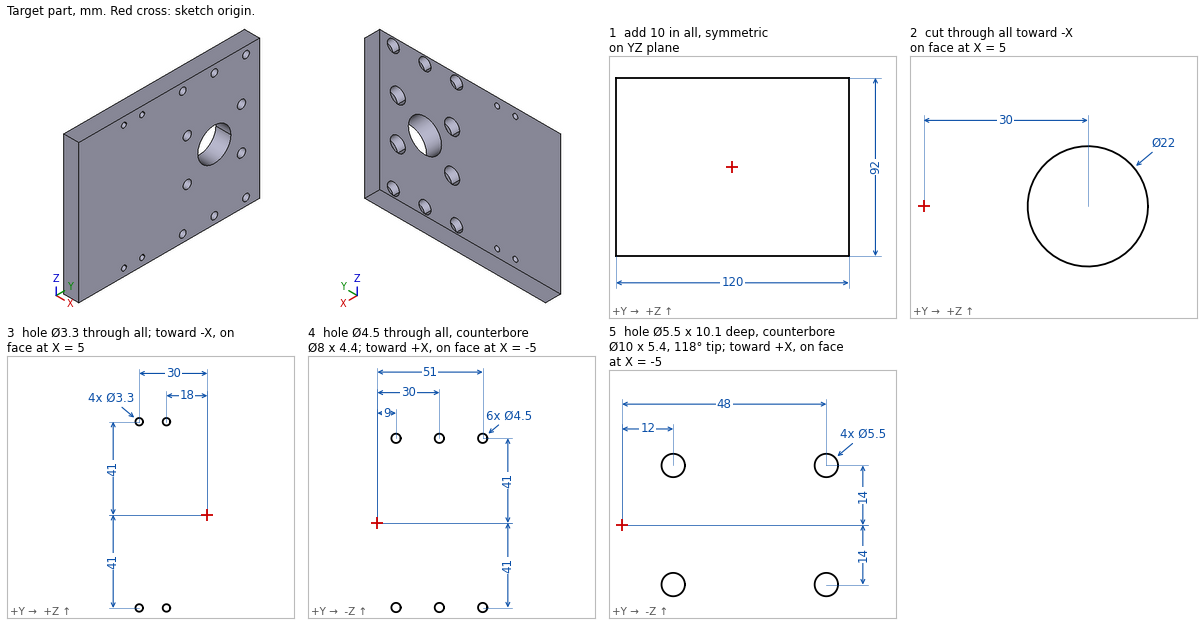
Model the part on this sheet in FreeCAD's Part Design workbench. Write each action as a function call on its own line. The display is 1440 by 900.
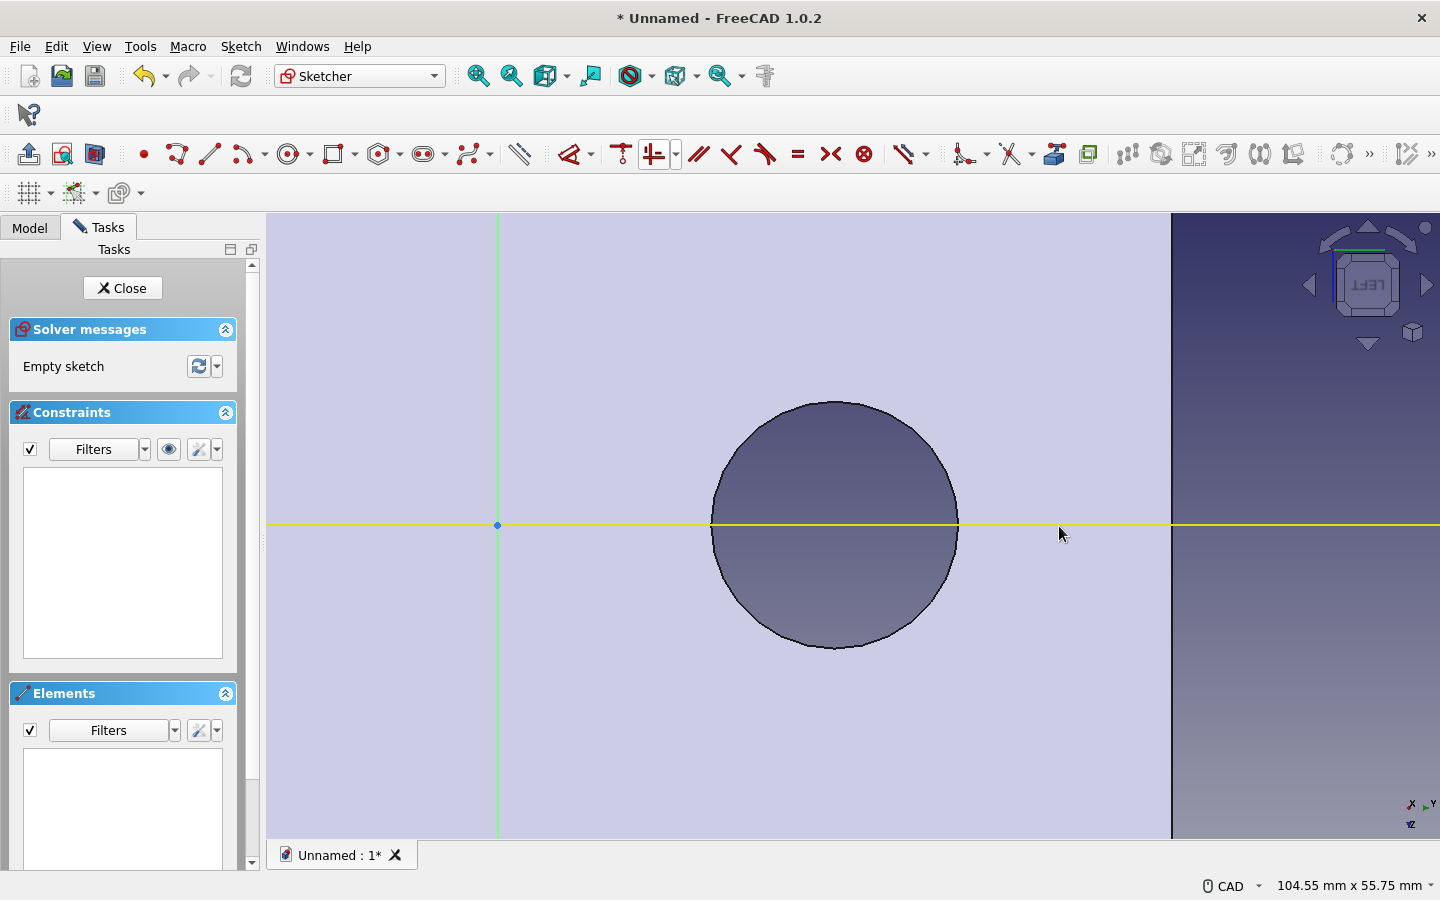
click(288, 154)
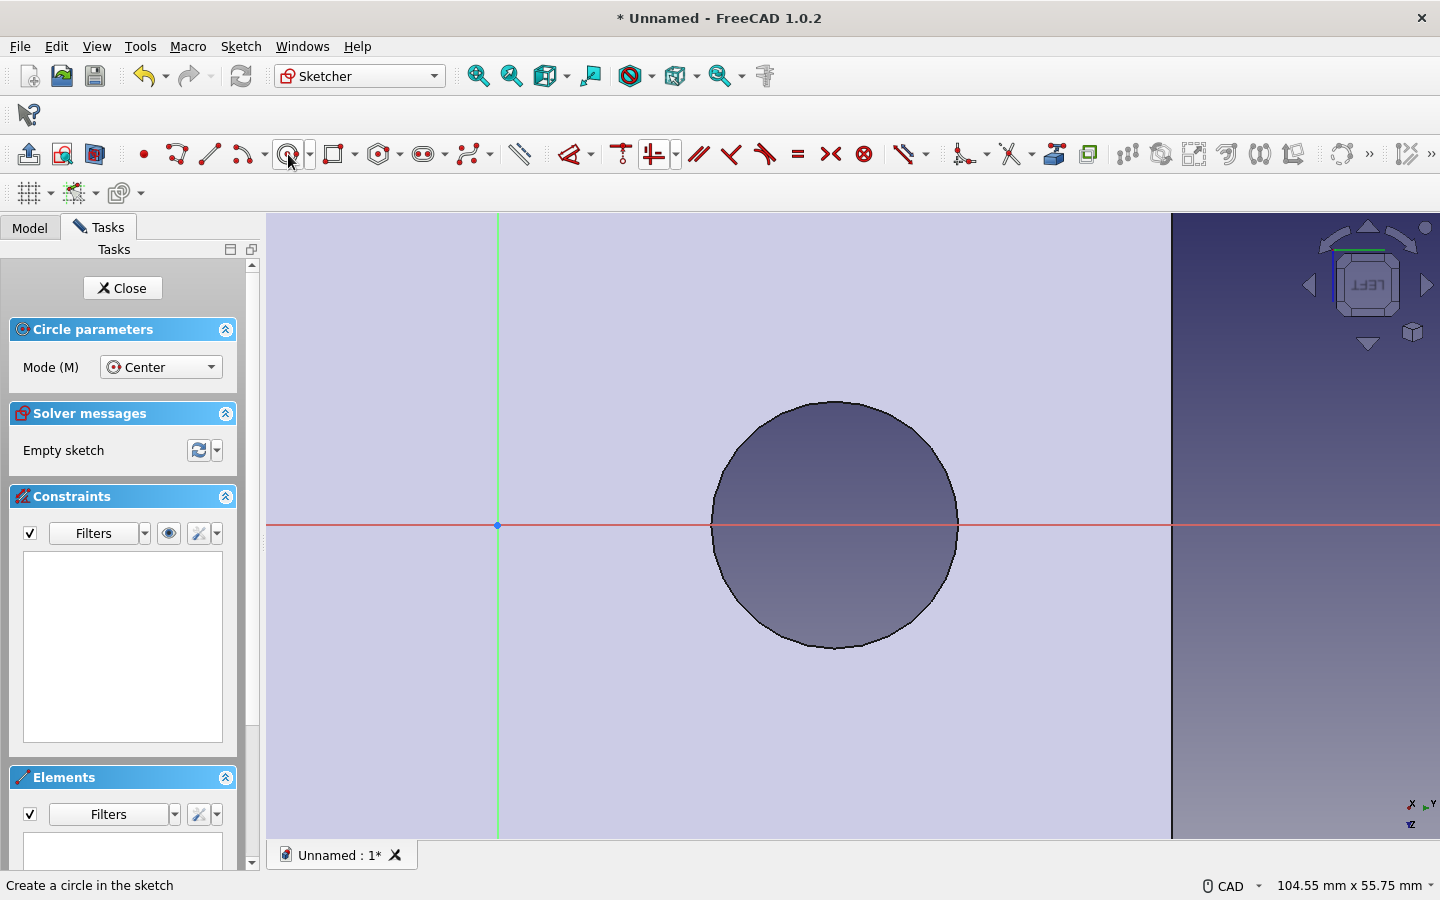
click(1037, 368)
click(1059, 346)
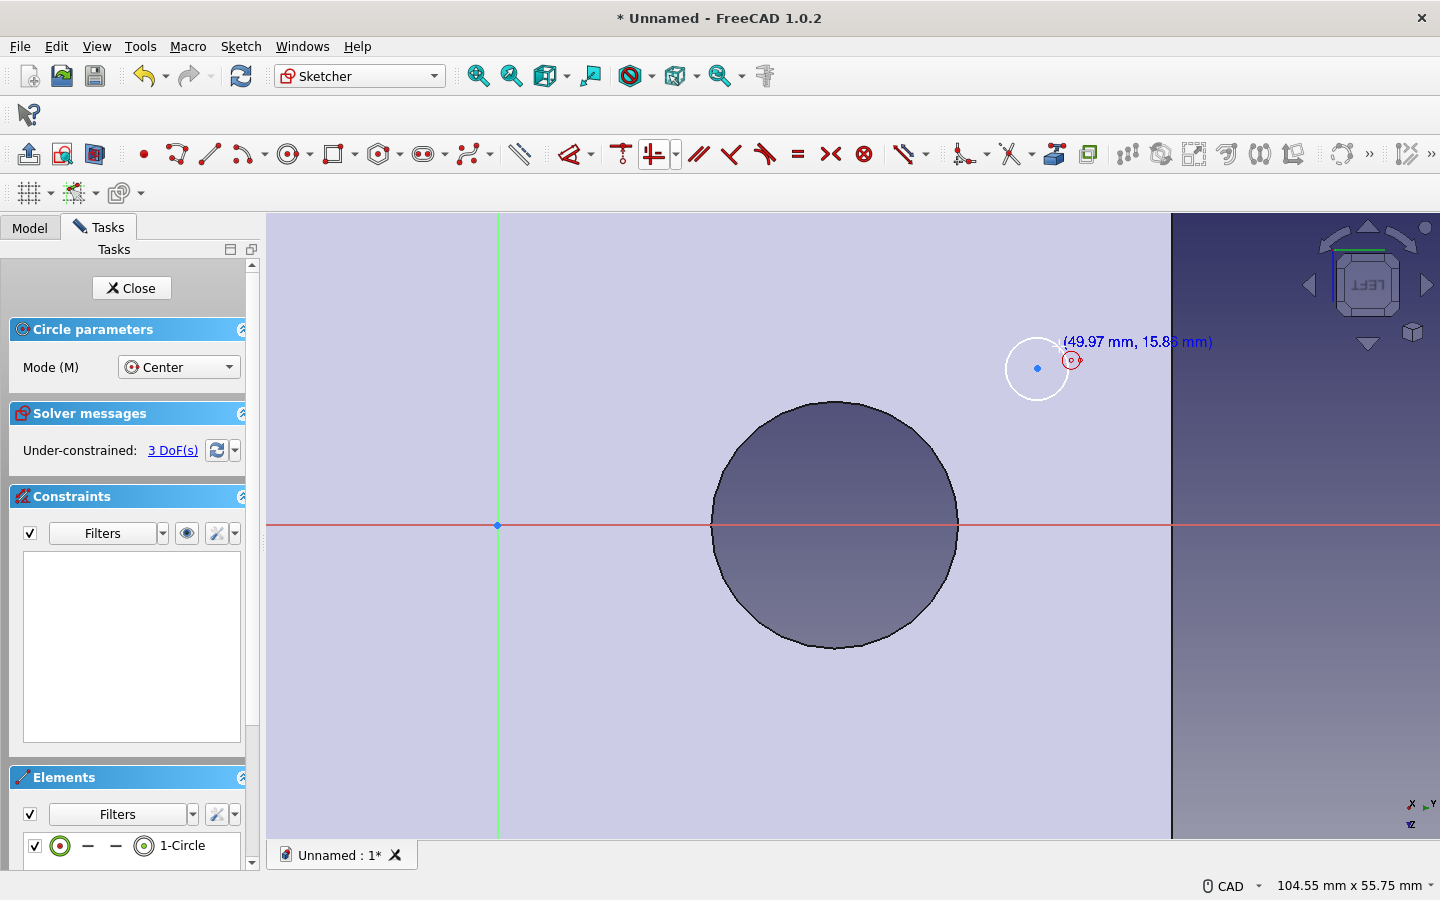
click(1037, 682)
click(1059, 661)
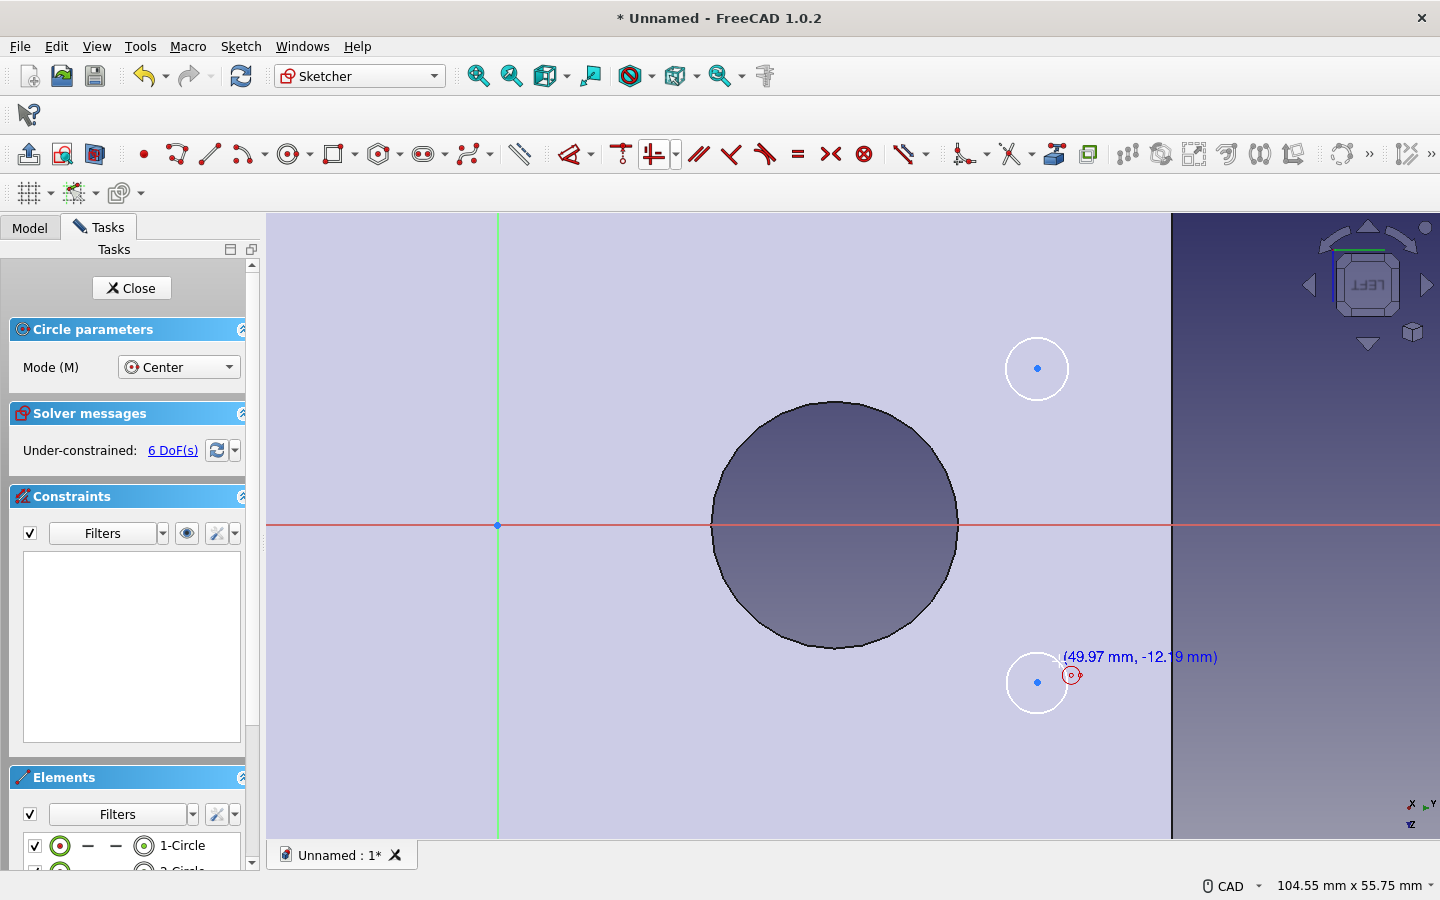
click(633, 368)
click(654, 346)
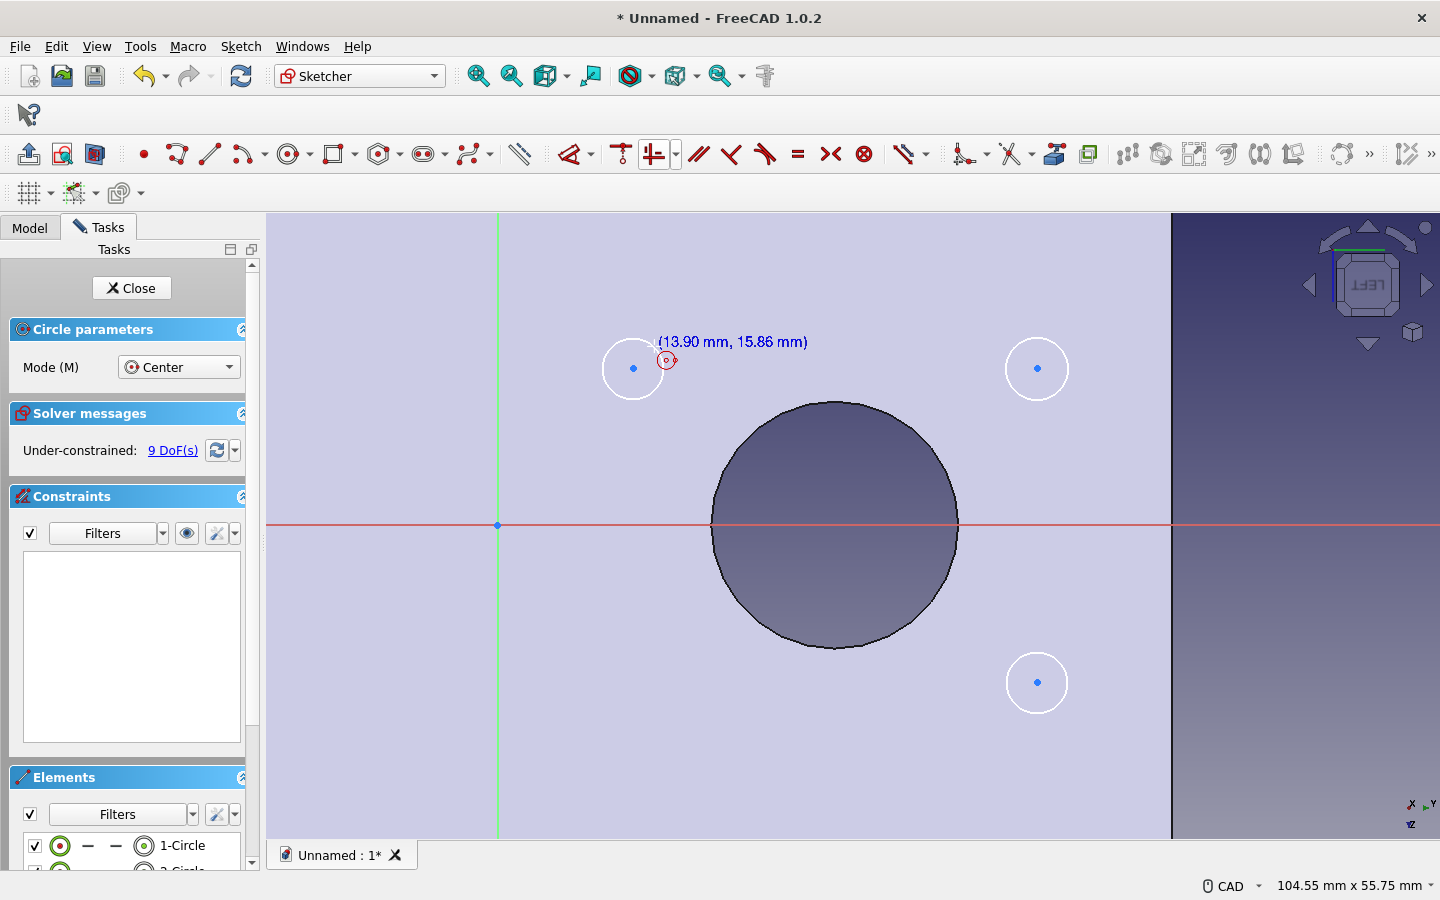
click(633, 682)
click(654, 661)
key(Escape)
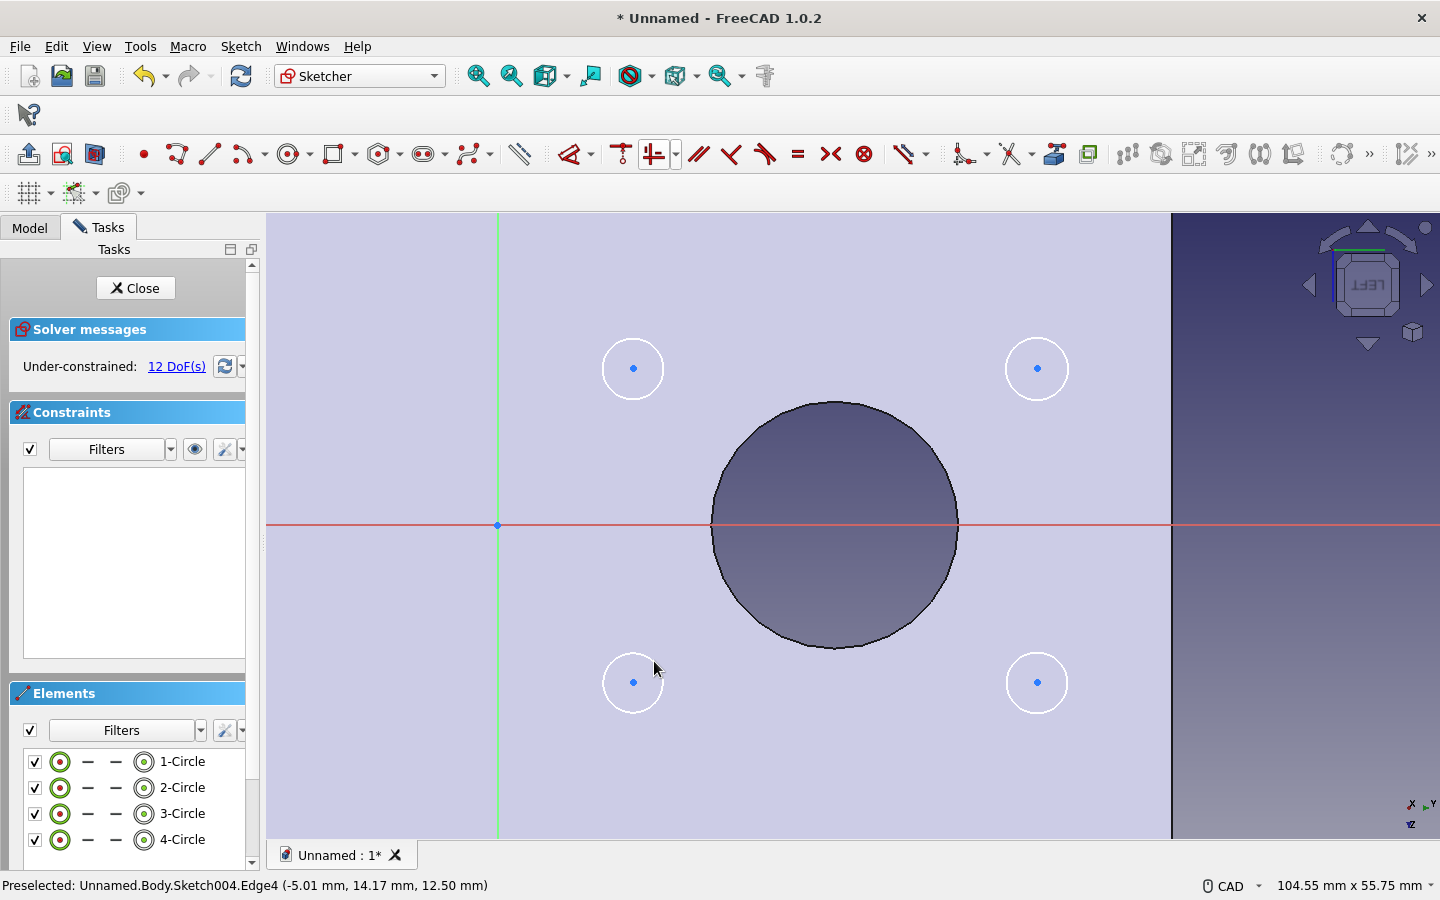
click(1059, 347)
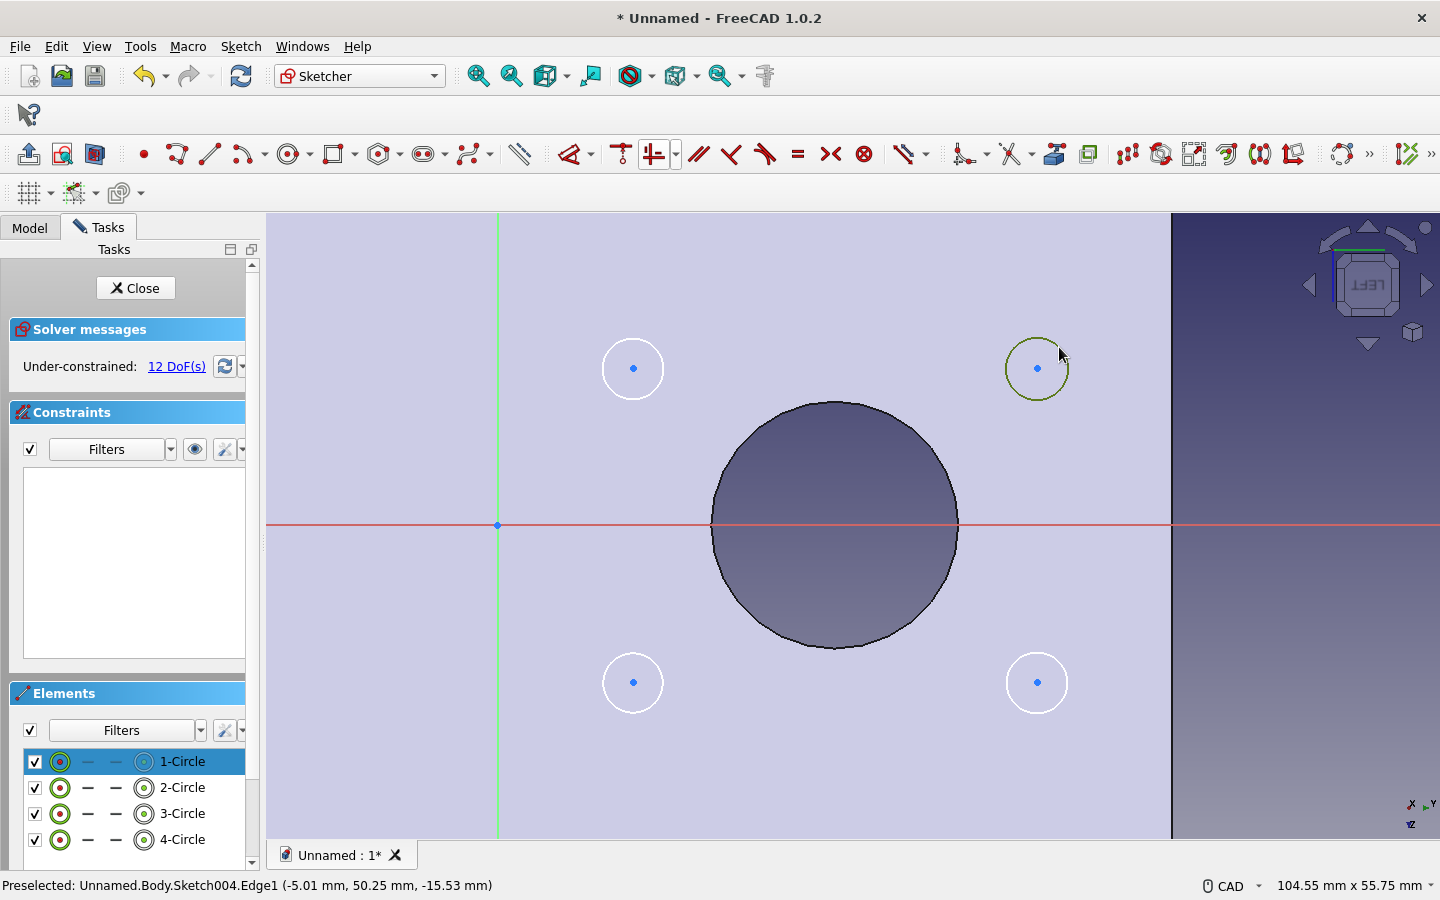
click(1058, 661)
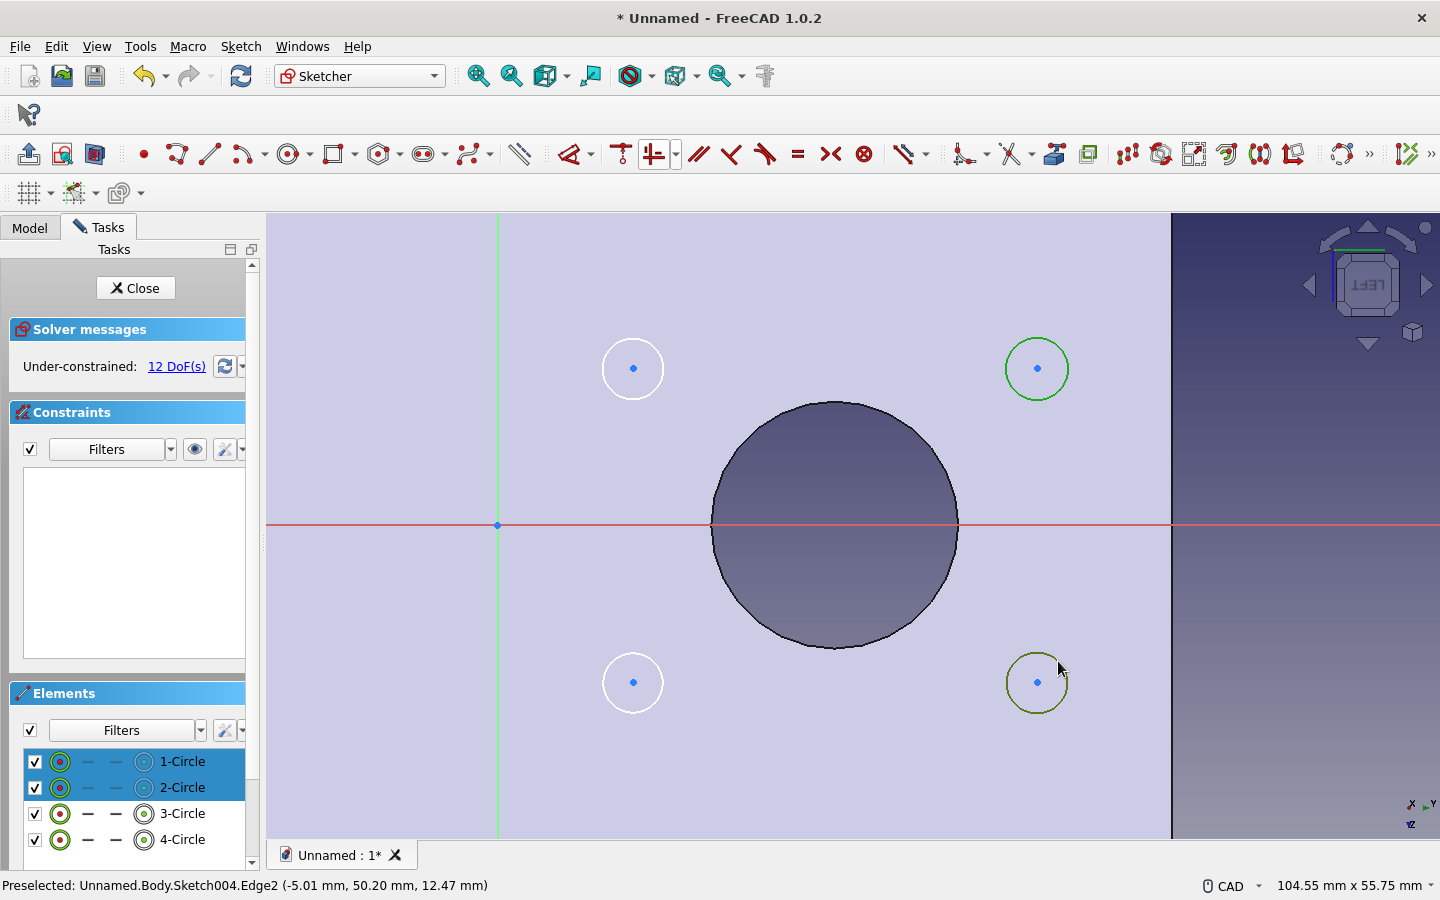
click(654, 347)